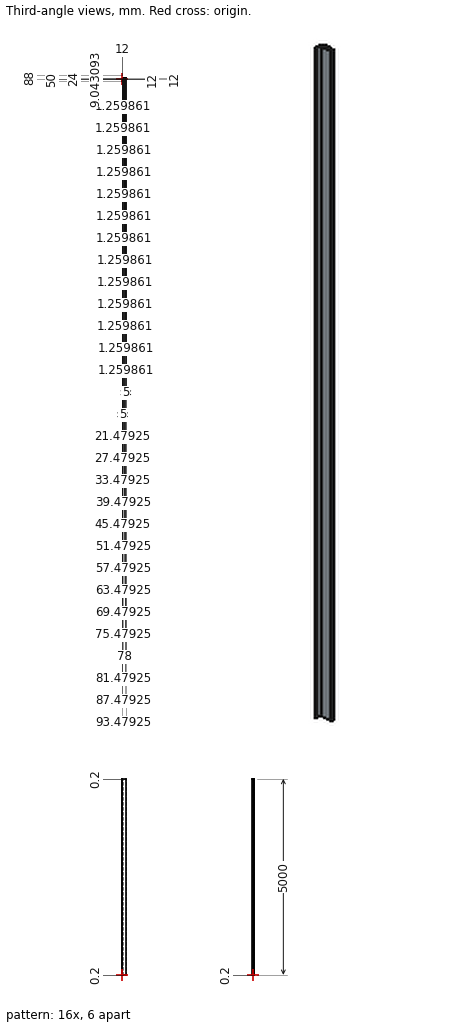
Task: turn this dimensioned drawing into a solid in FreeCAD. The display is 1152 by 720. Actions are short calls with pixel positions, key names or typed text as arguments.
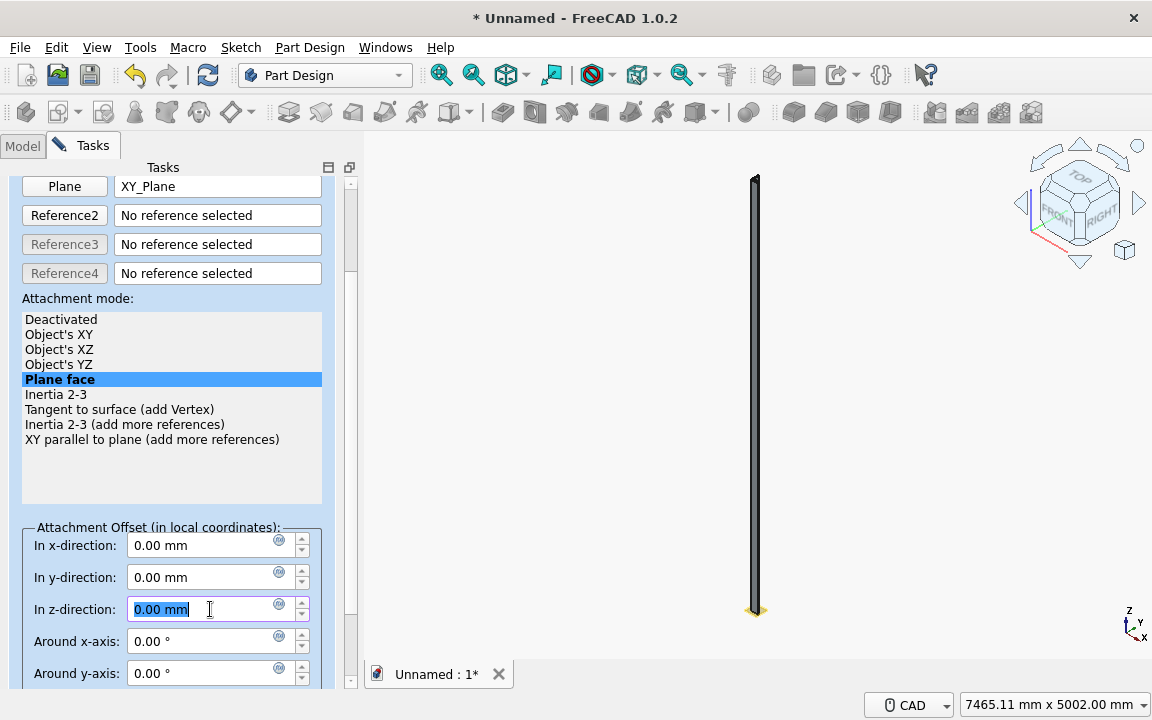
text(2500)
key(Tab)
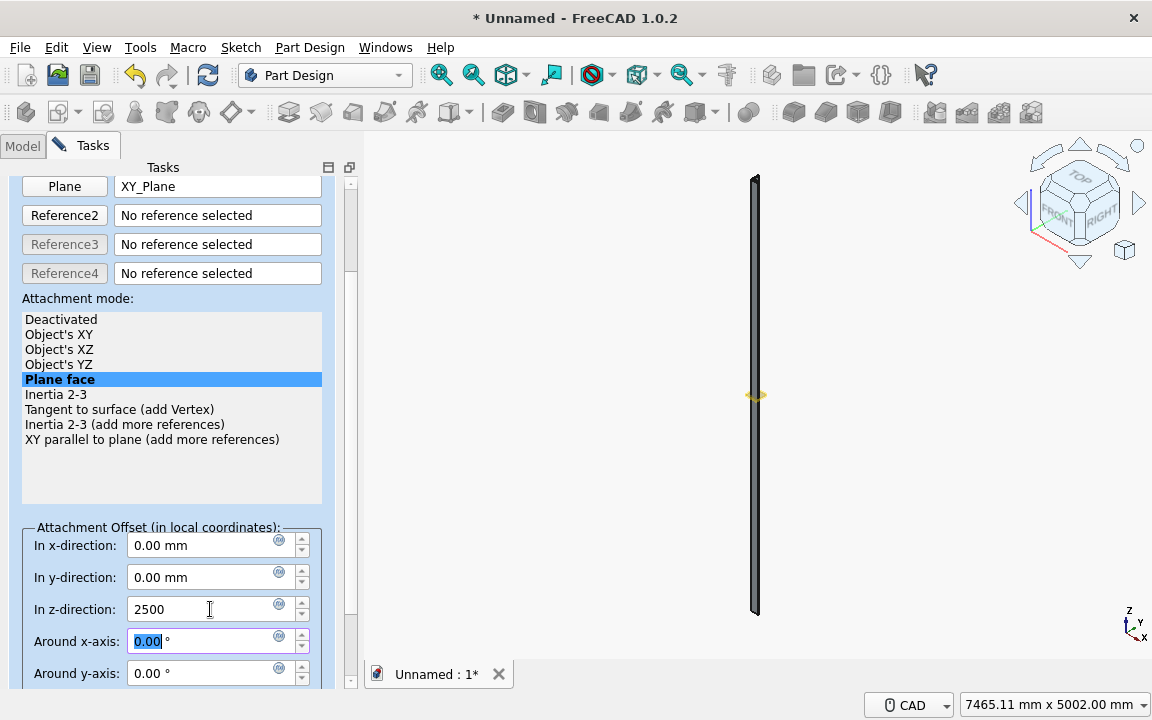
scroll(351, 432, up, 3)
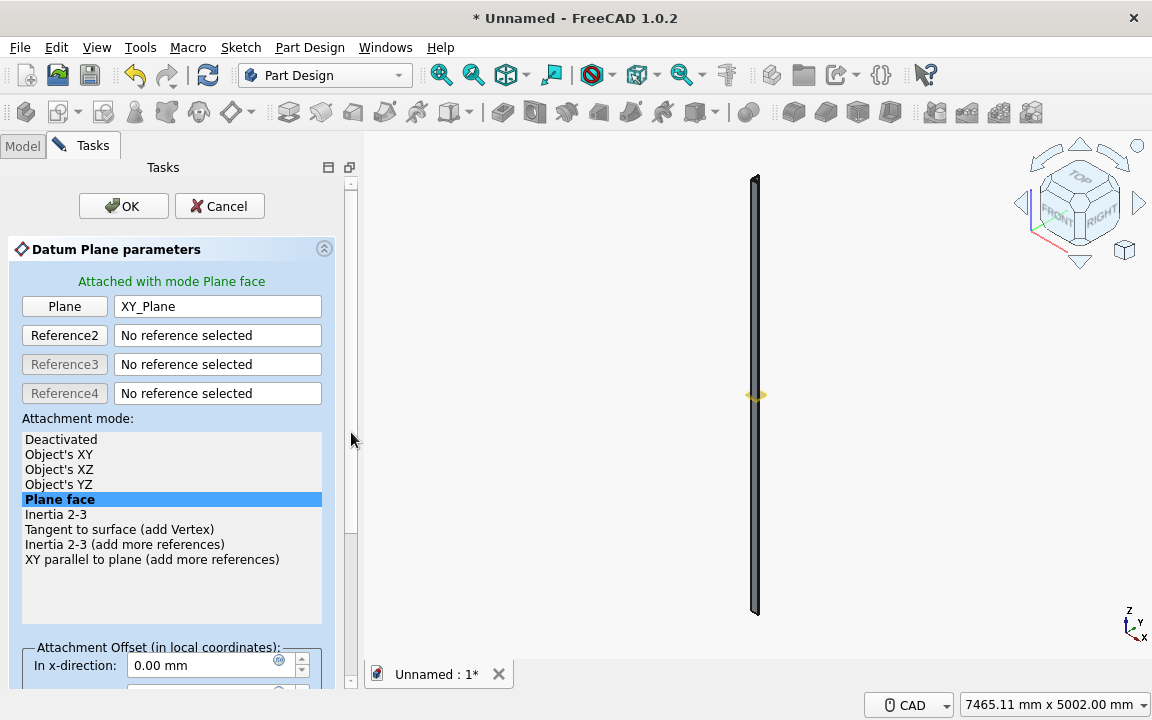
click(124, 206)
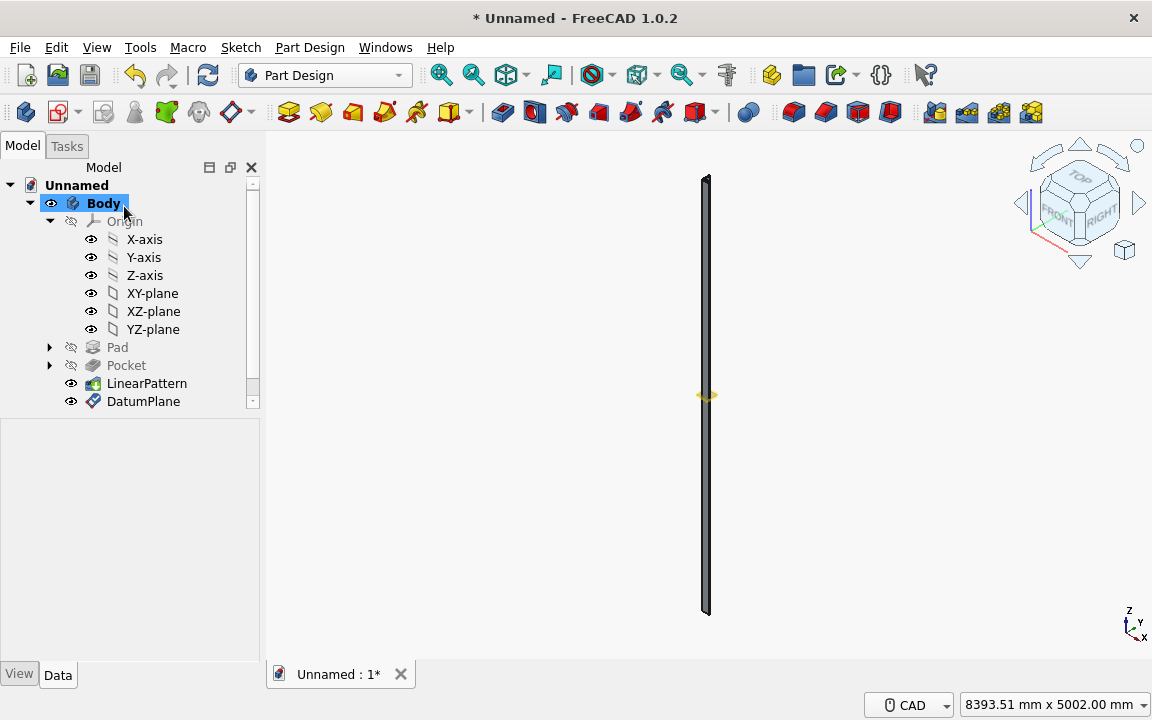
click(116, 365)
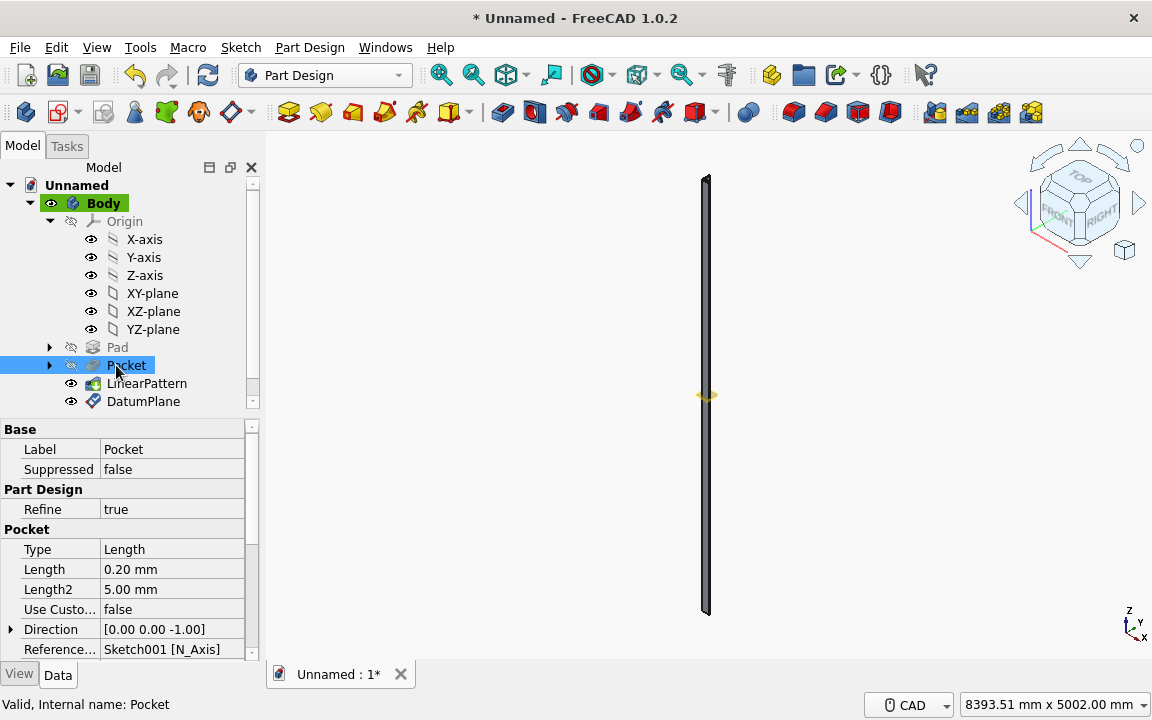
click(936, 112)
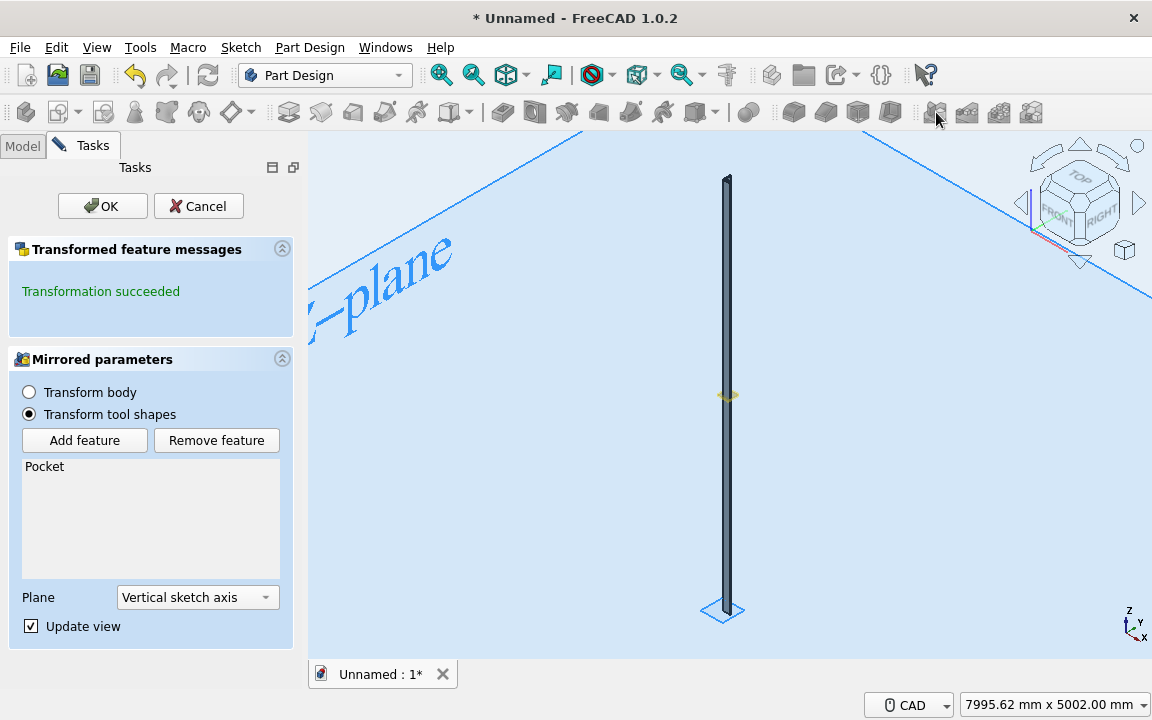
click(198, 598)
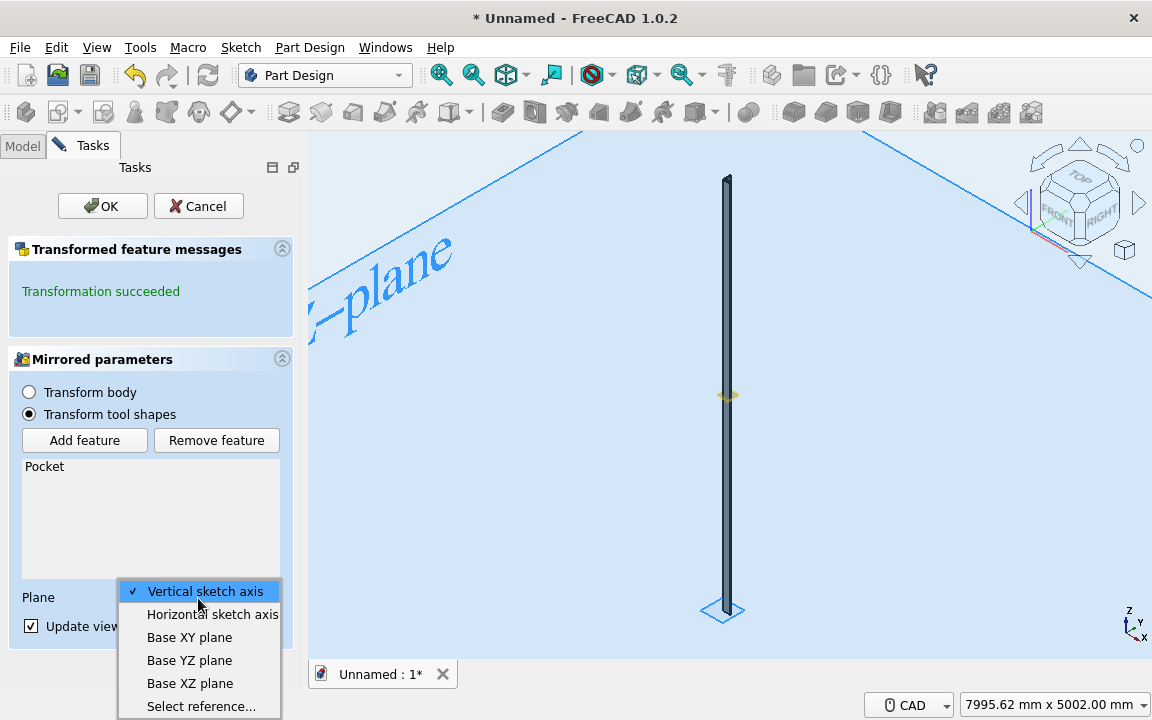
click(198, 706)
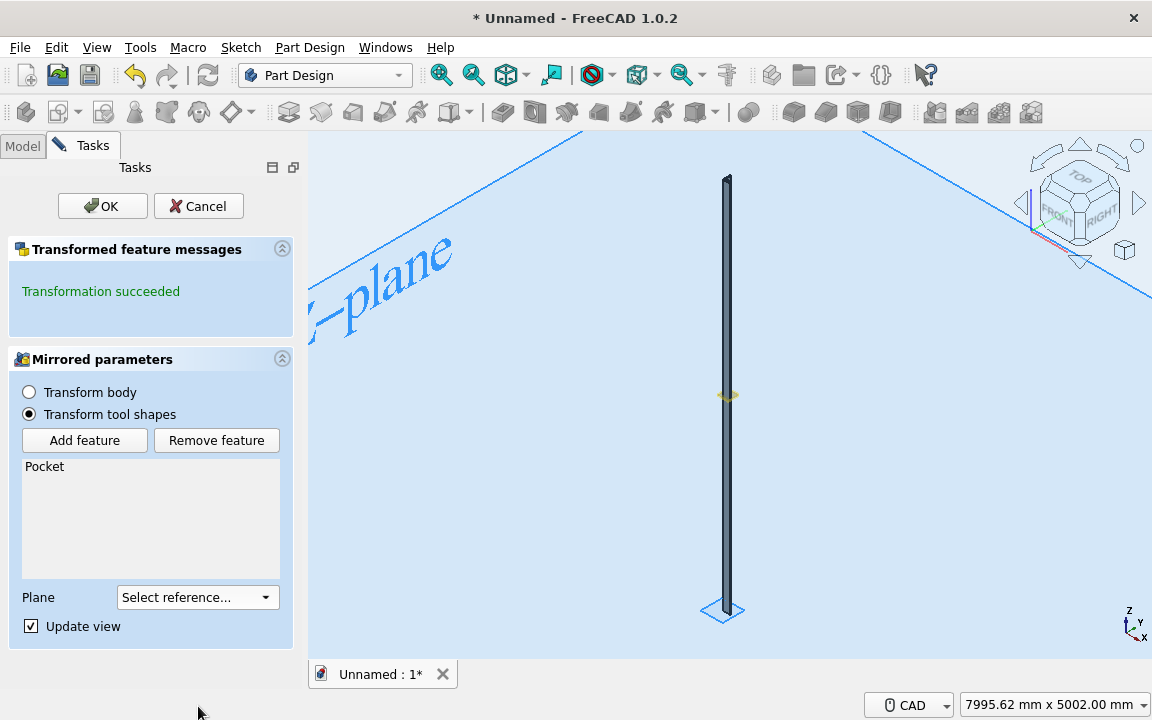
click(23, 145)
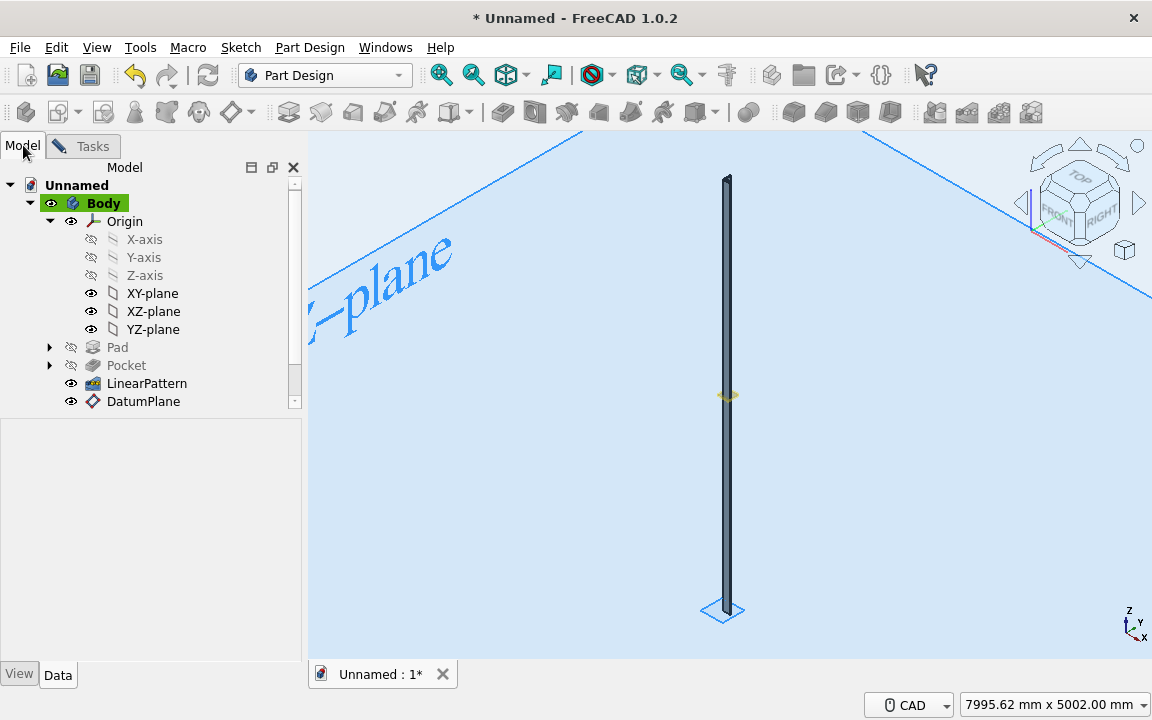
click(116, 401)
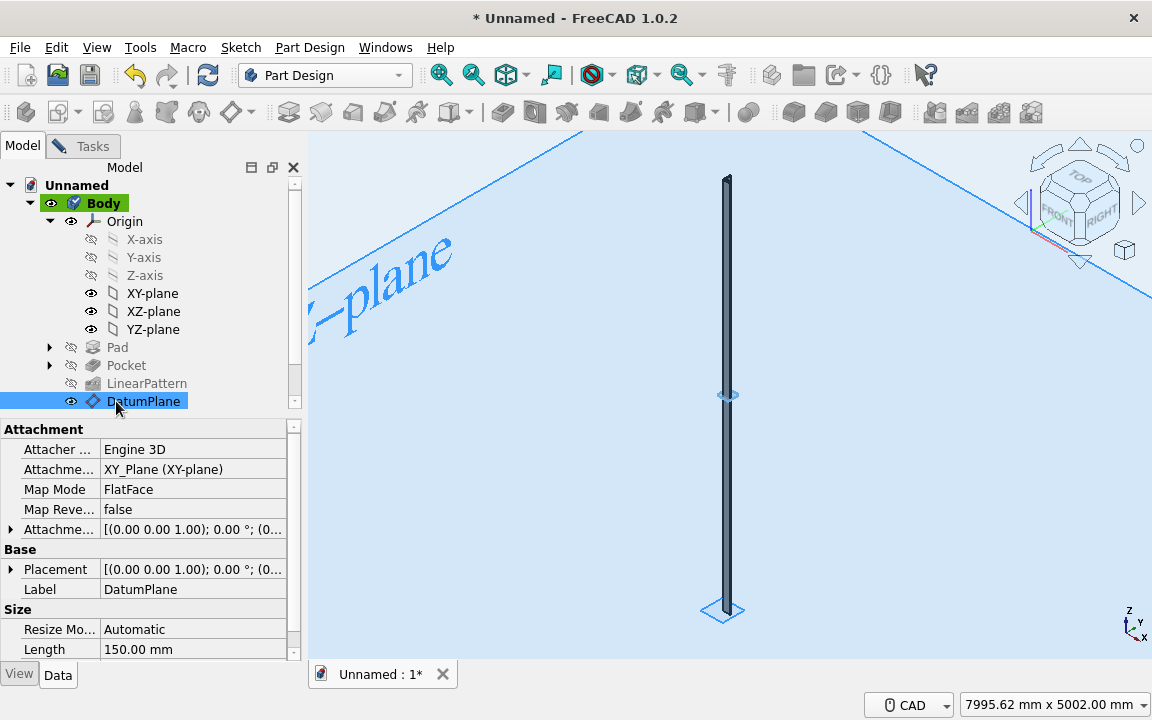
click(84, 145)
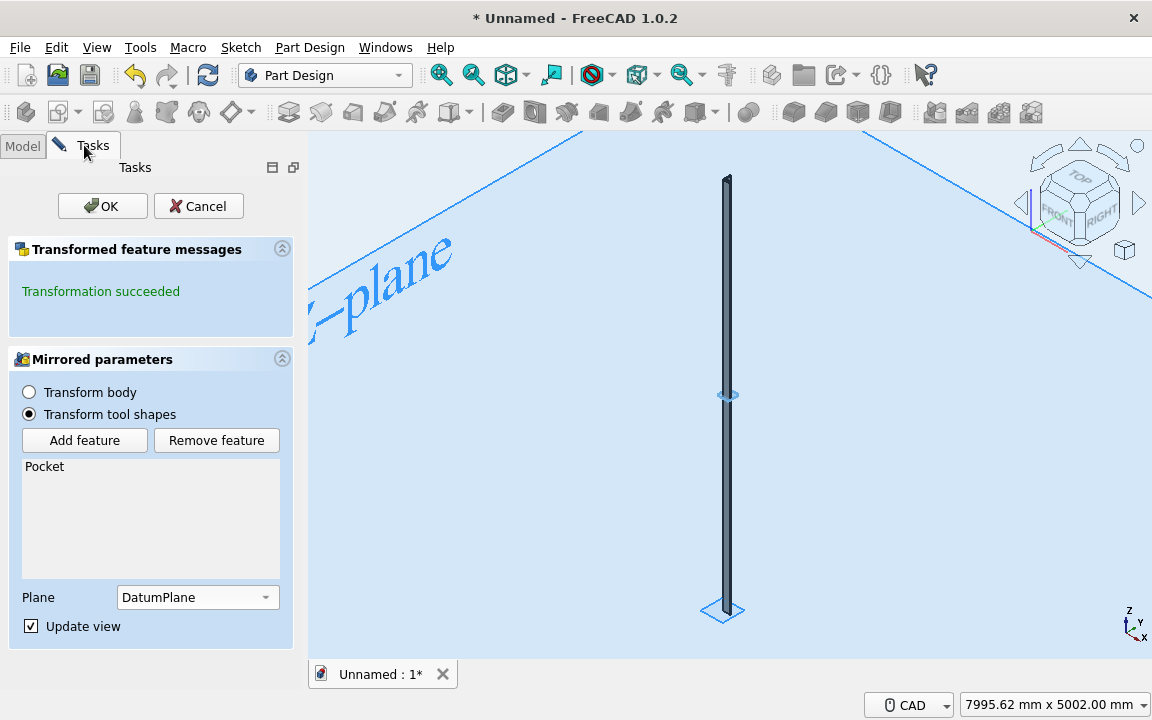
click(103, 206)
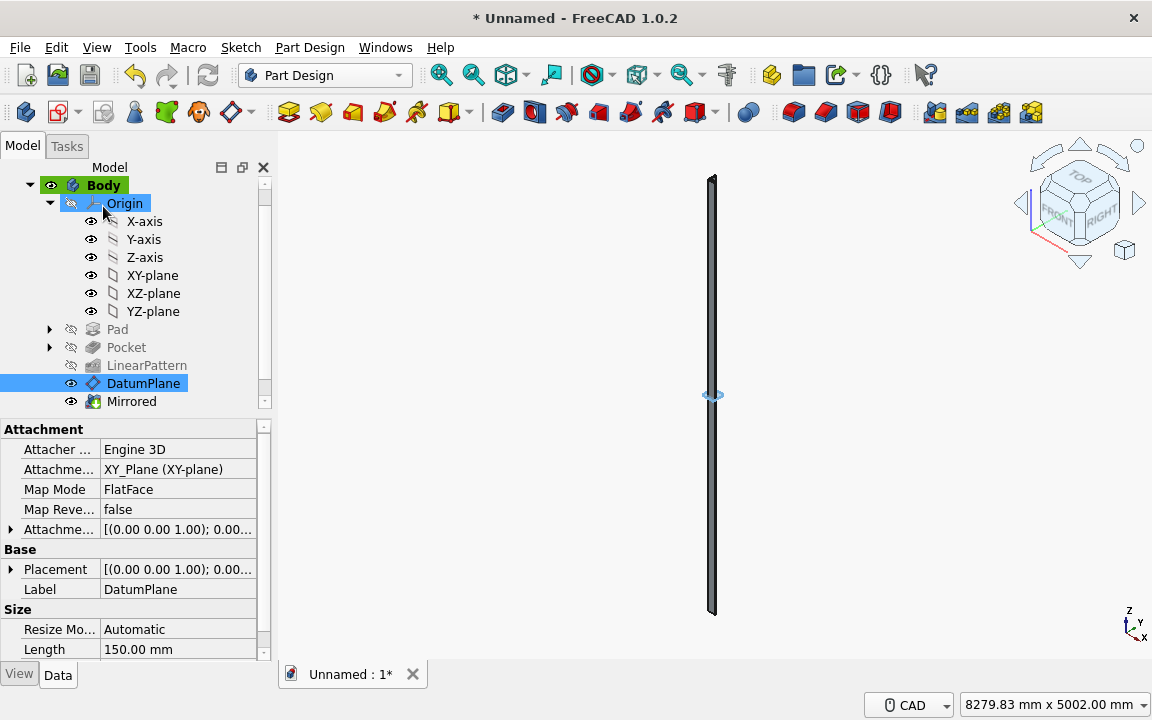
click(116, 383)
key(space)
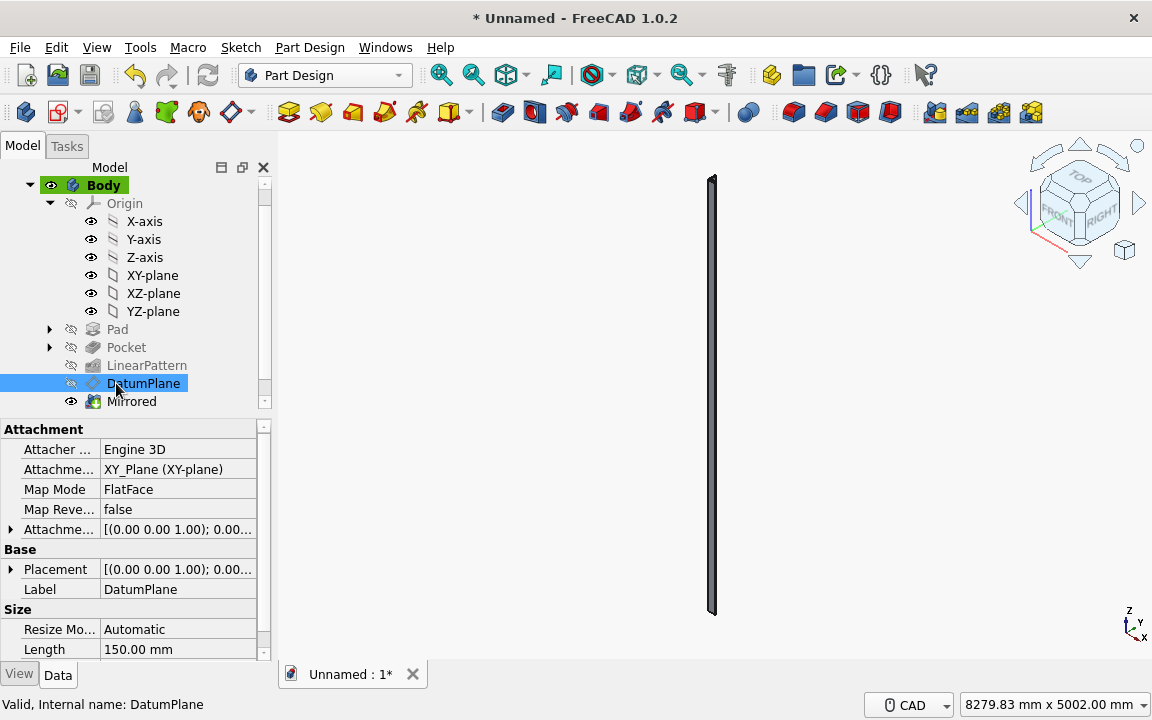
key(5)